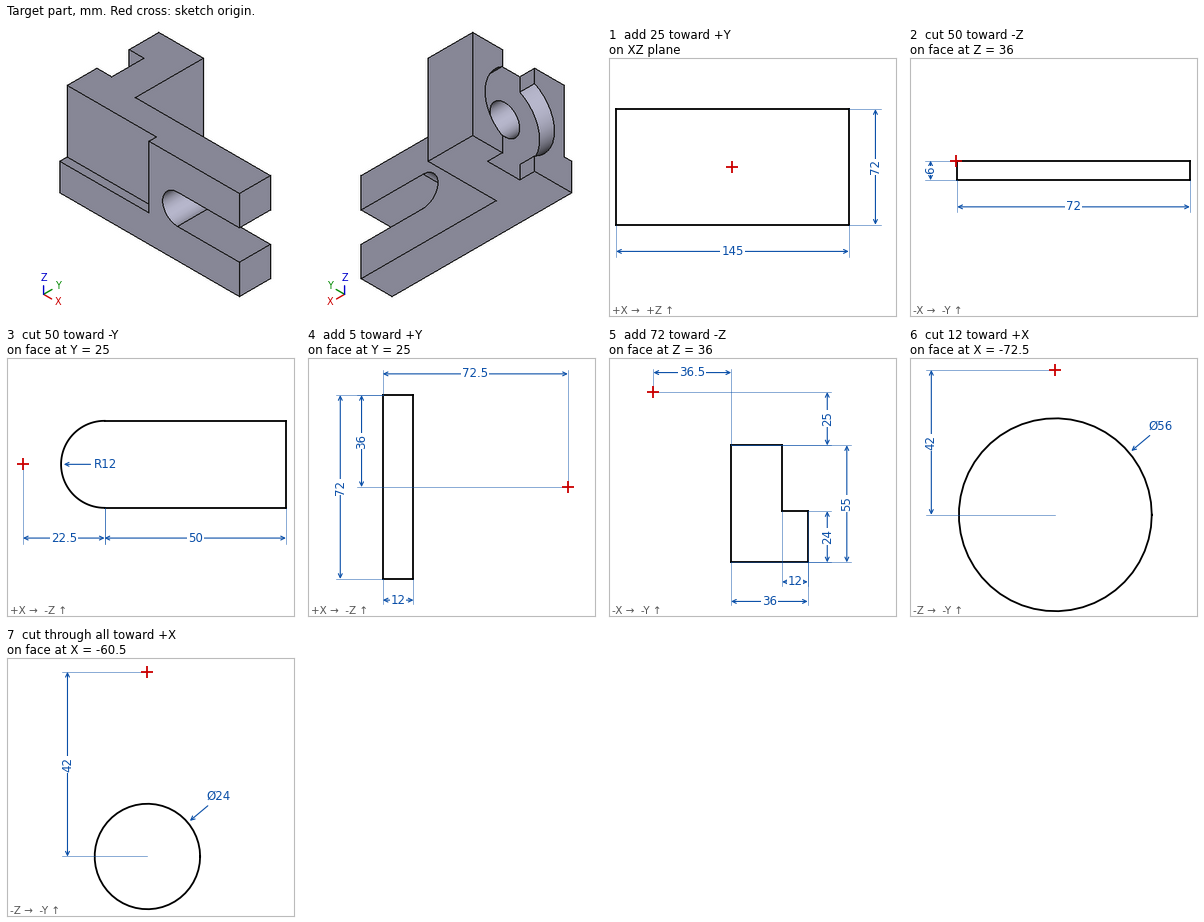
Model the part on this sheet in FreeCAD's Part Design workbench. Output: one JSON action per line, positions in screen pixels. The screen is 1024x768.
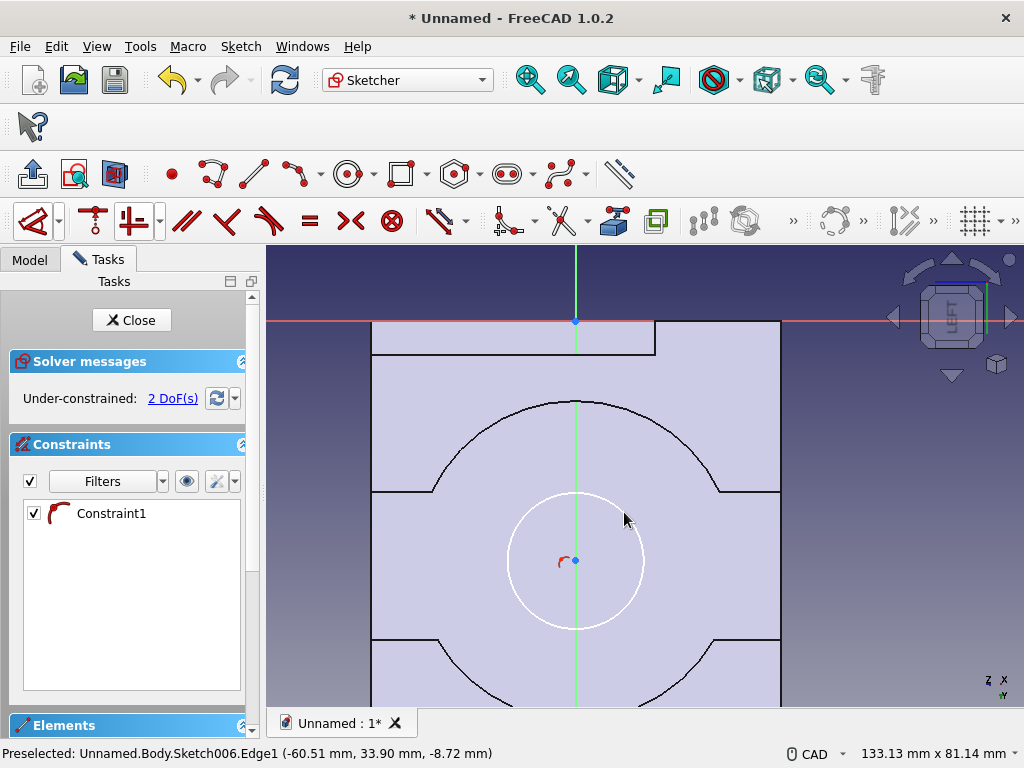
{"action": "left_click", "coordinate": [624, 513]}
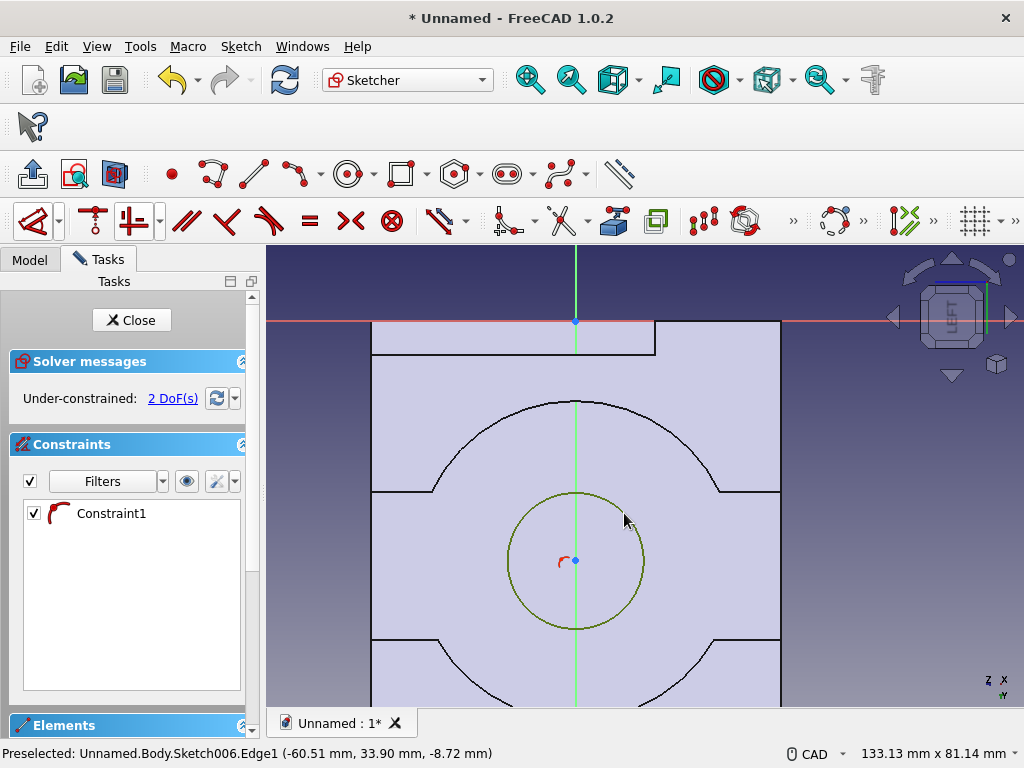
{"action": "left_click", "coordinate": [58, 222]}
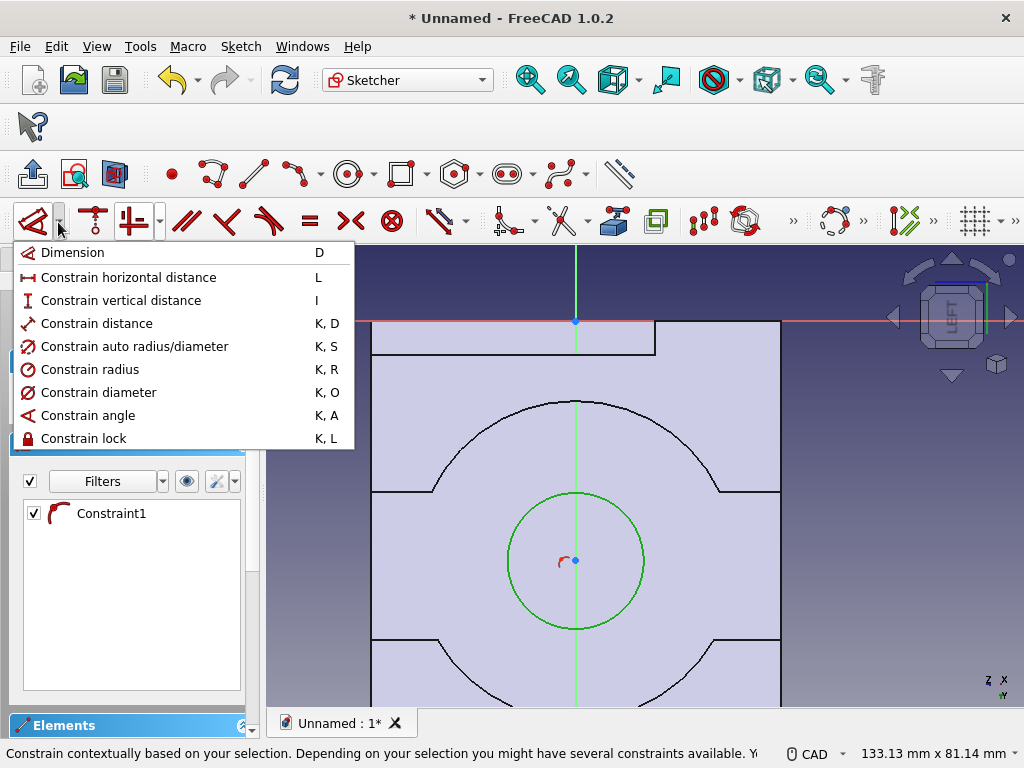
{"action": "left_click", "coordinate": [184, 392]}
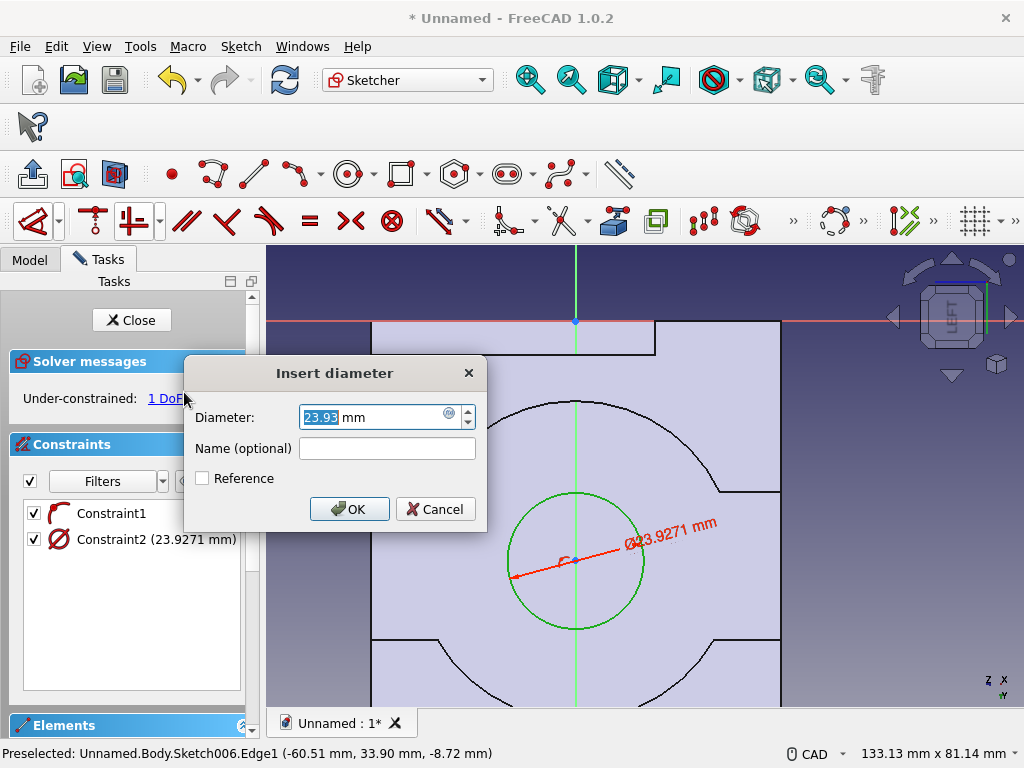
{"action": "type", "text": "24"}
{"action": "key", "text": "Return"}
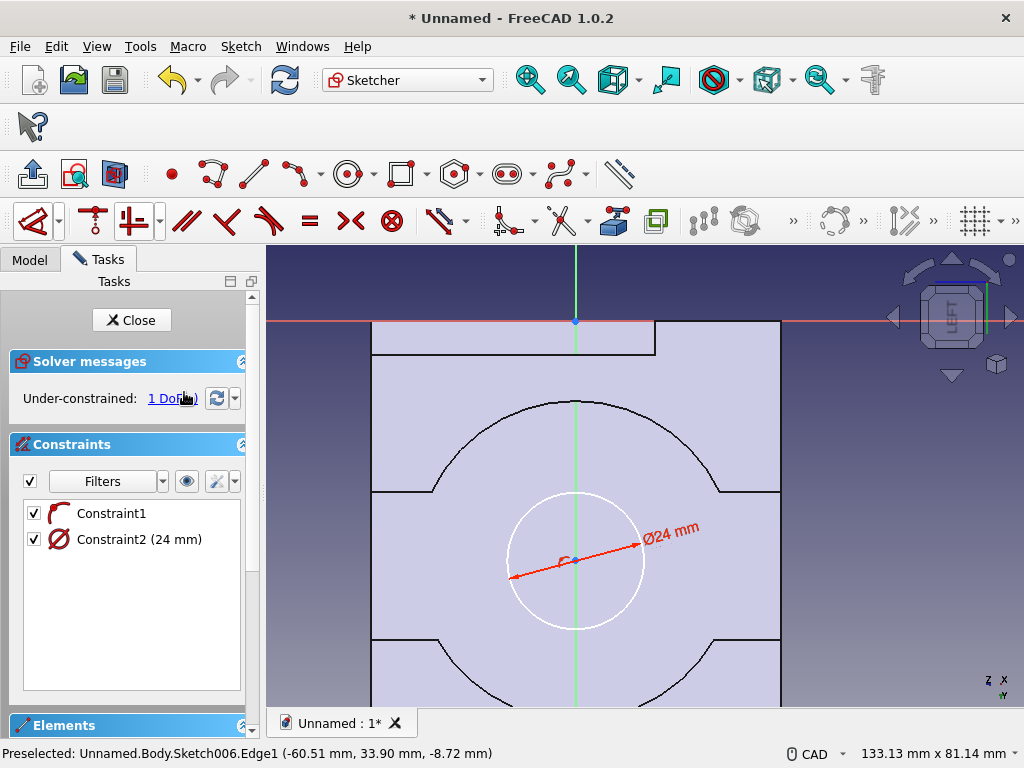
{"action": "left_click", "coordinate": [576, 561]}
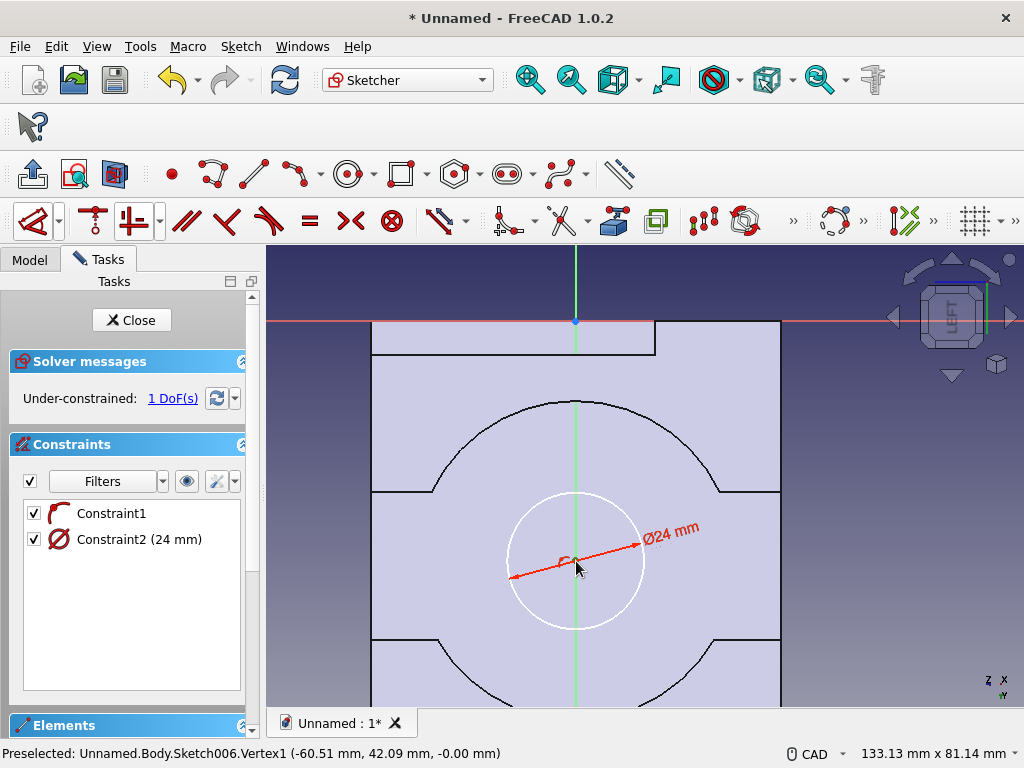
{"action": "left_click", "coordinate": [58, 222]}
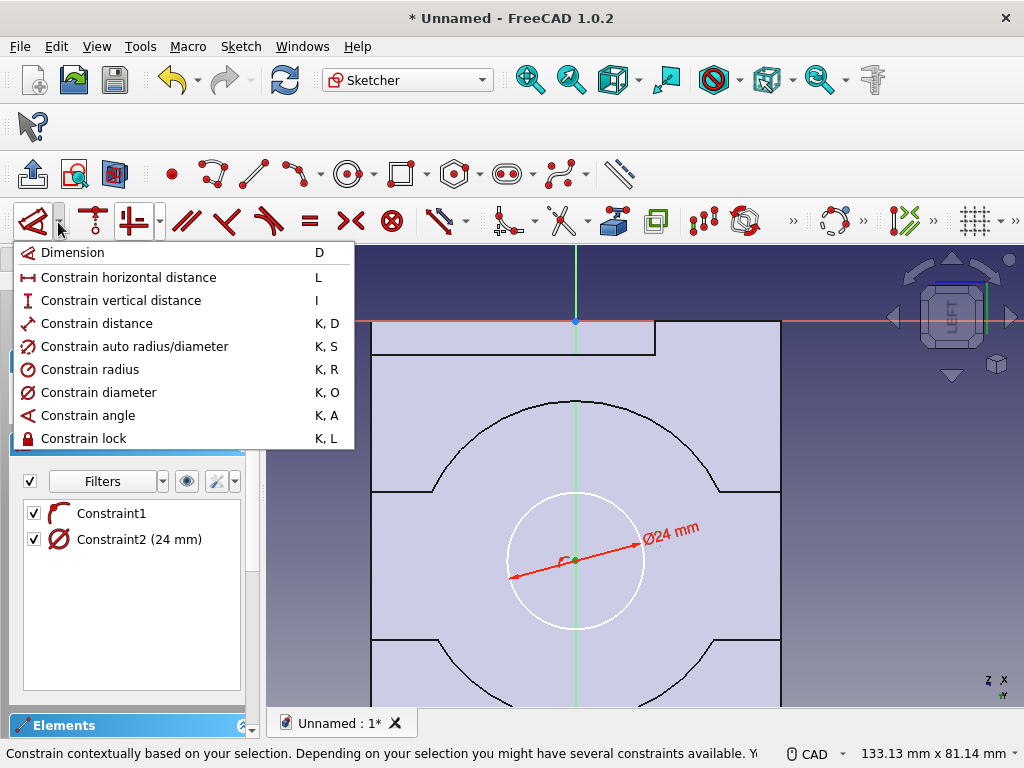
{"action": "left_click", "coordinate": [184, 300]}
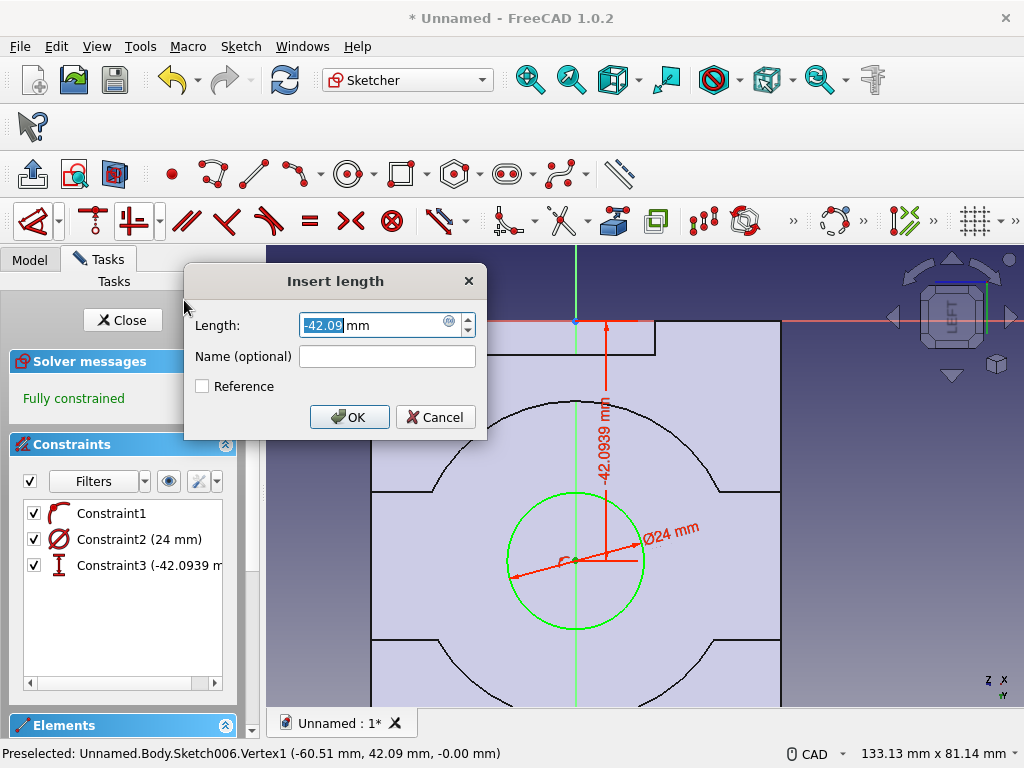
{"action": "type", "text": "-42"}
{"action": "key", "text": "Return"}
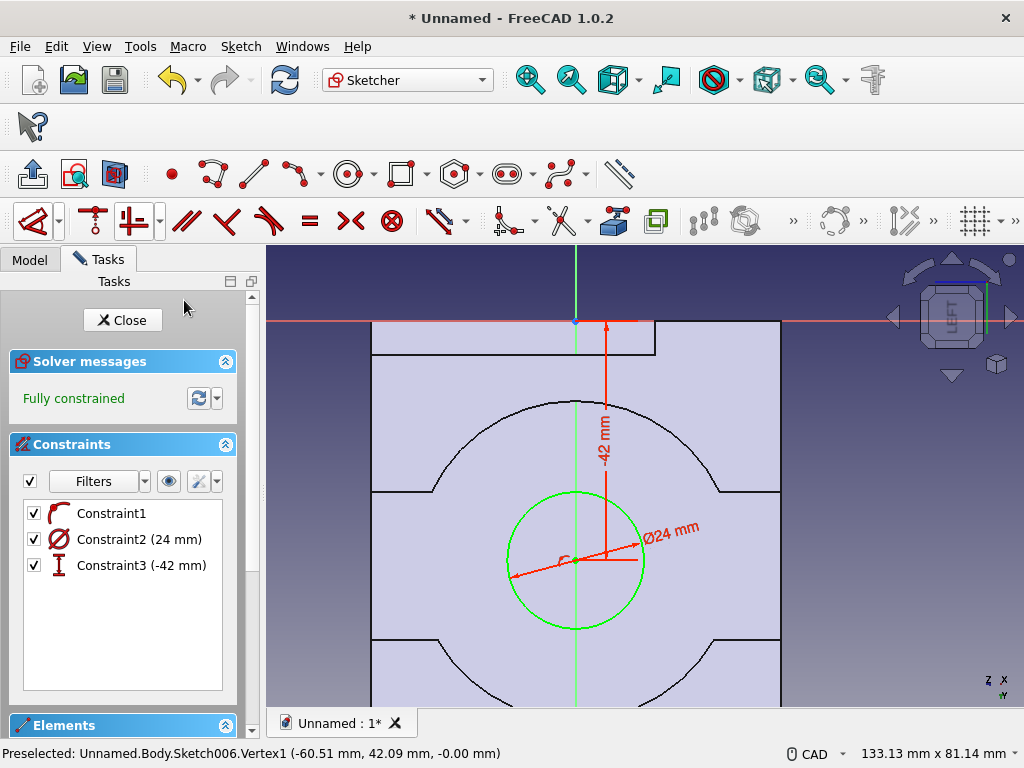
{"action": "left_click", "coordinate": [123, 320]}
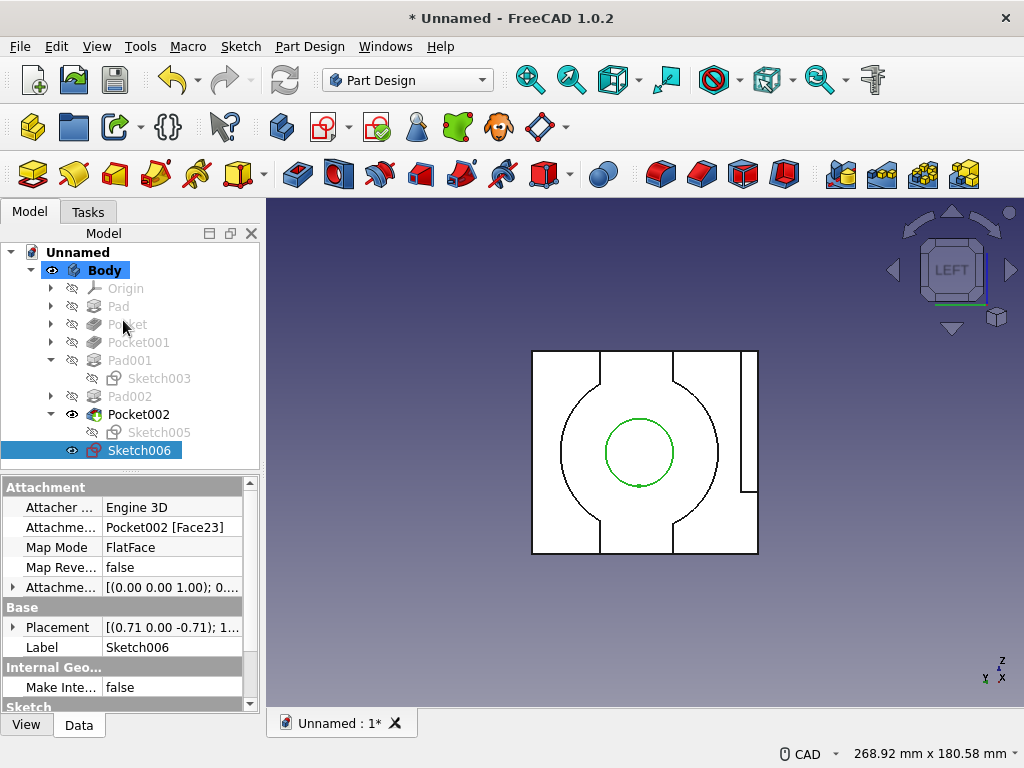
{"action": "left_click", "coordinate": [298, 174]}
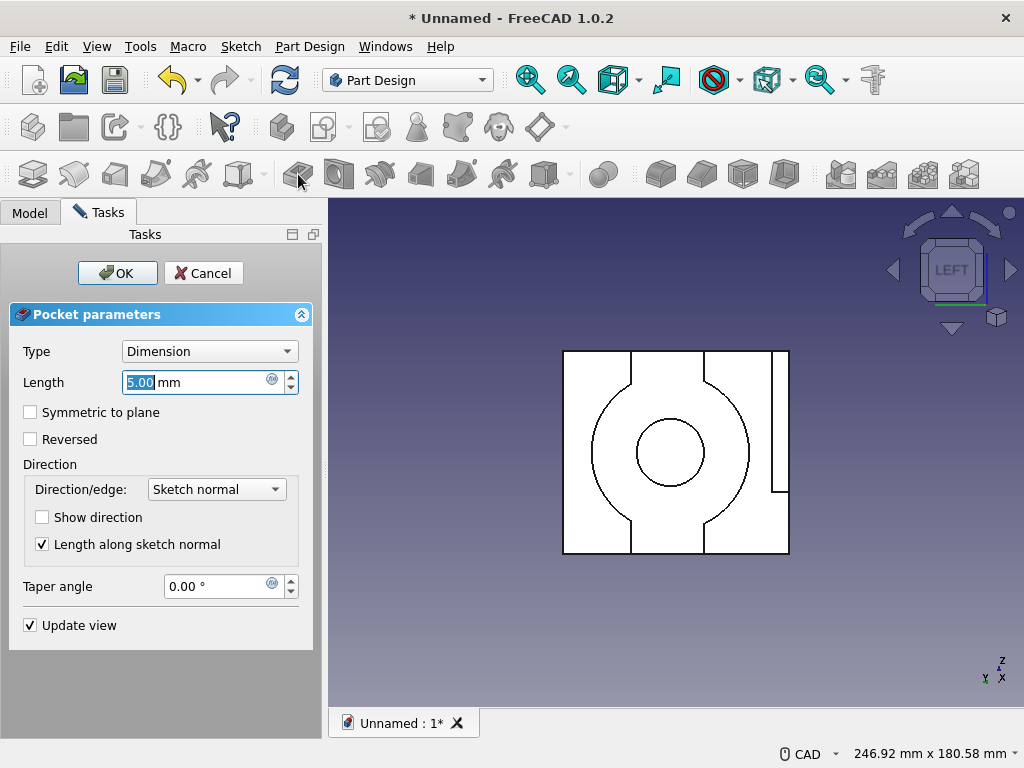
{"action": "left_click", "coordinate": [210, 352]}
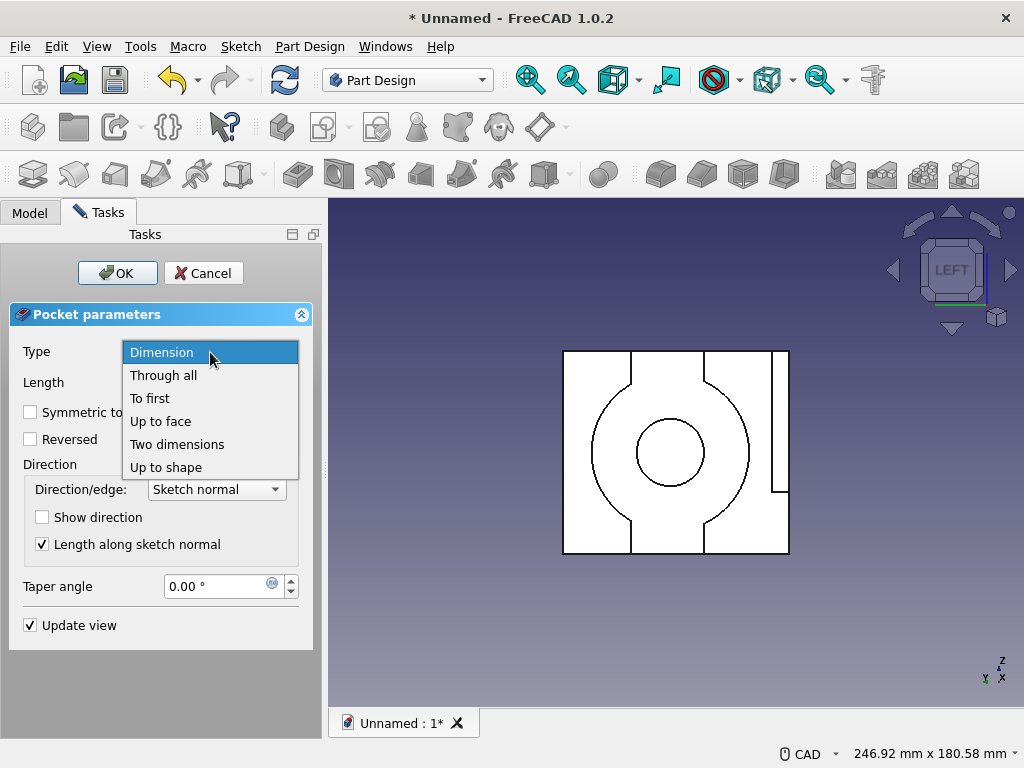
{"action": "left_click", "coordinate": [208, 376]}